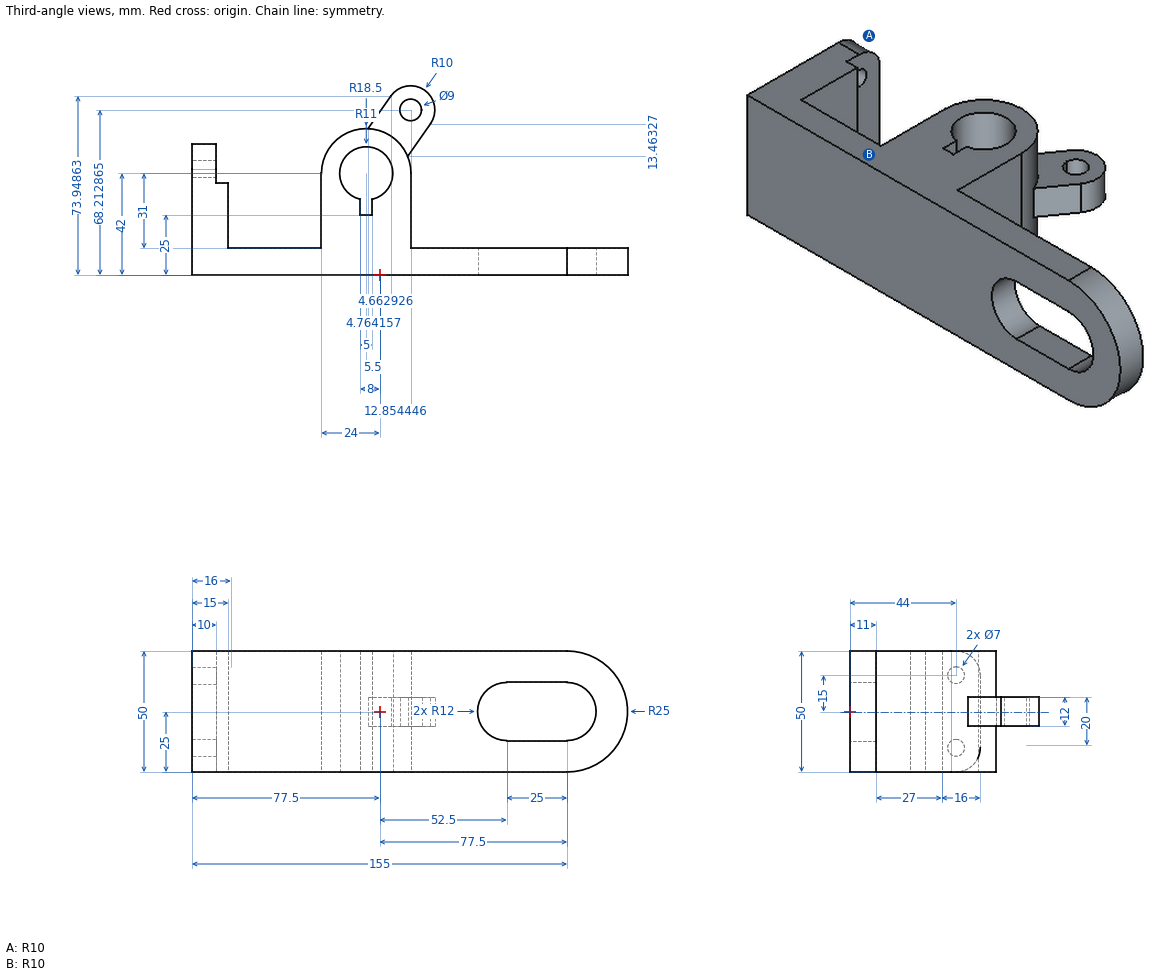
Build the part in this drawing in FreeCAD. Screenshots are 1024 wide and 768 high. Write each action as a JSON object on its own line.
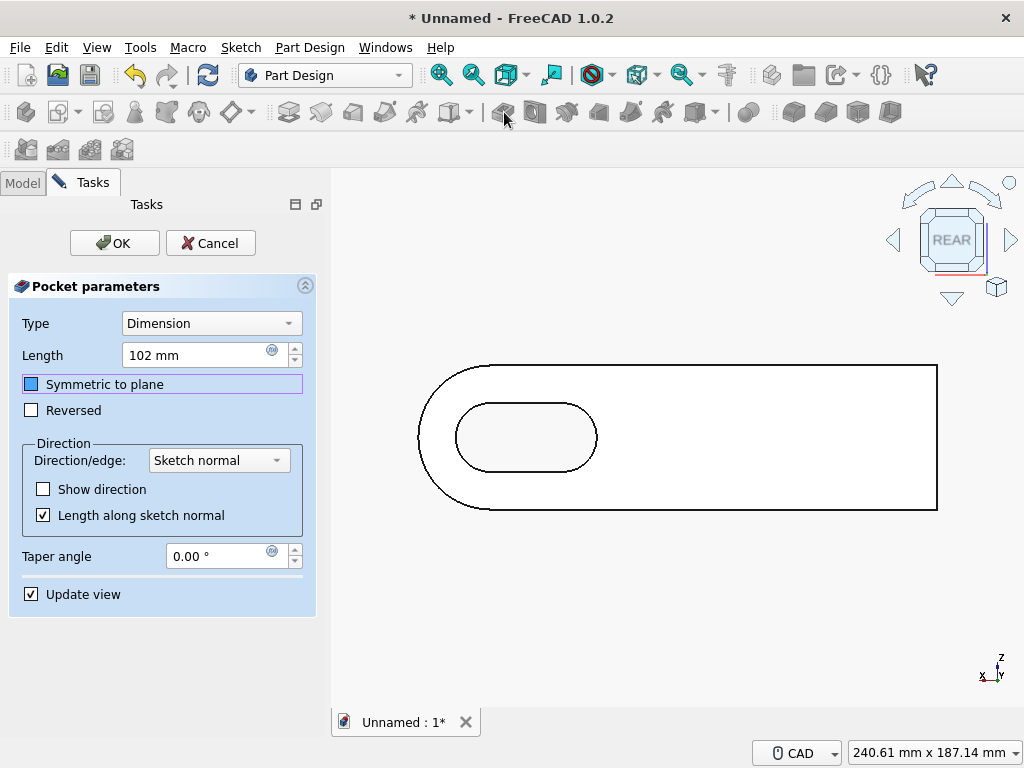
{"action": "left_click", "coordinate": [115, 243]}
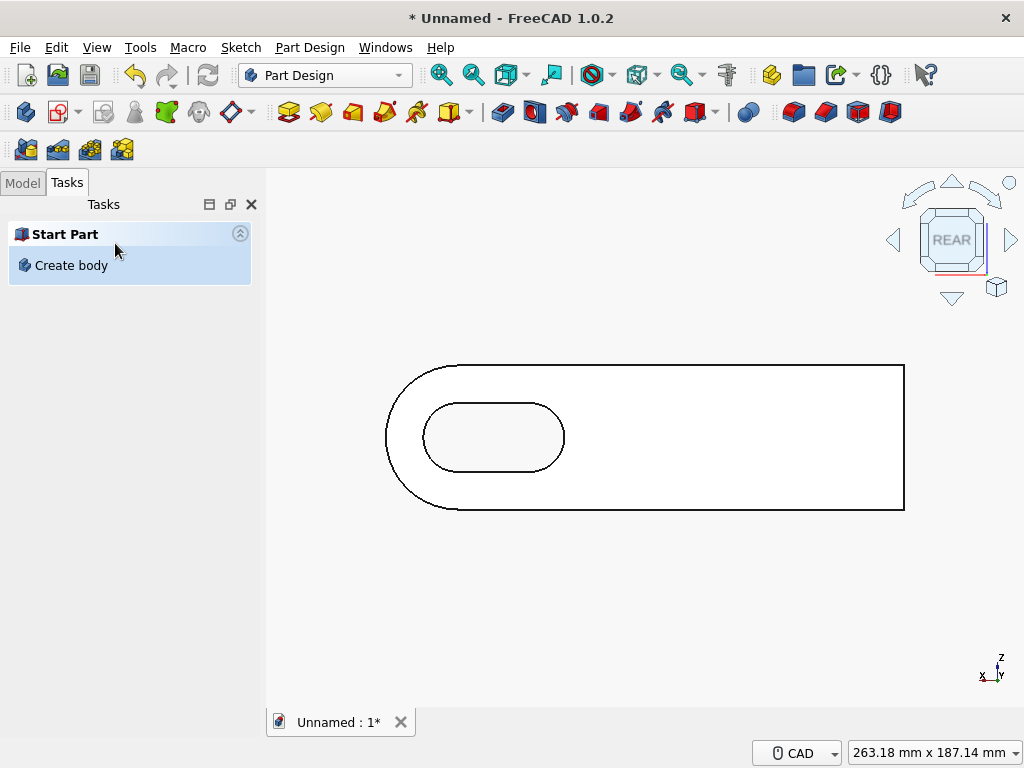
{"action": "key", "text": "0"}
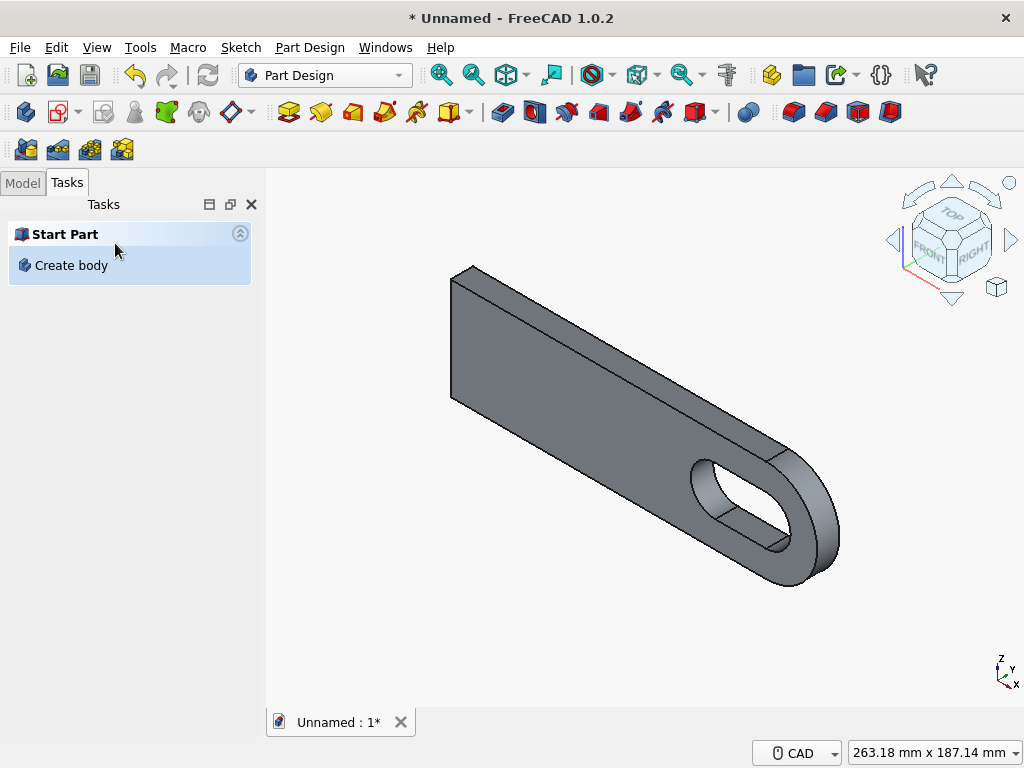
{"action": "left_click", "coordinate": [755, 441]}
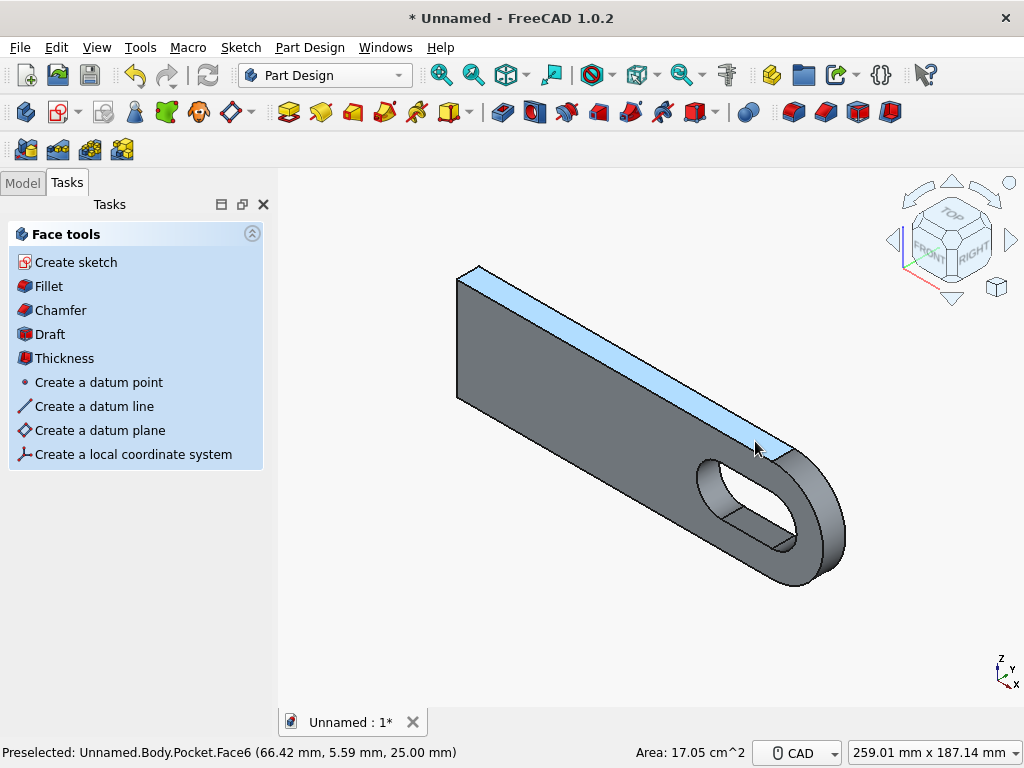
{"action": "left_click", "coordinate": [58, 112]}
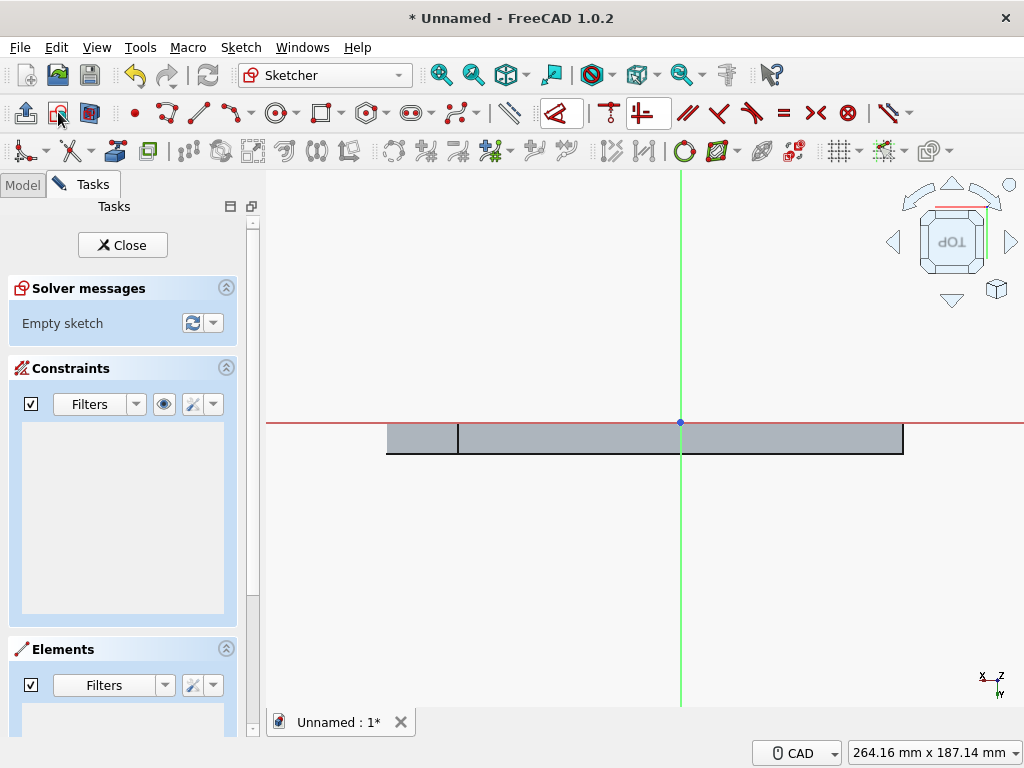
{"action": "scroll", "coordinate": [843, 596], "scroll_direction": "up", "scroll_amount": 3}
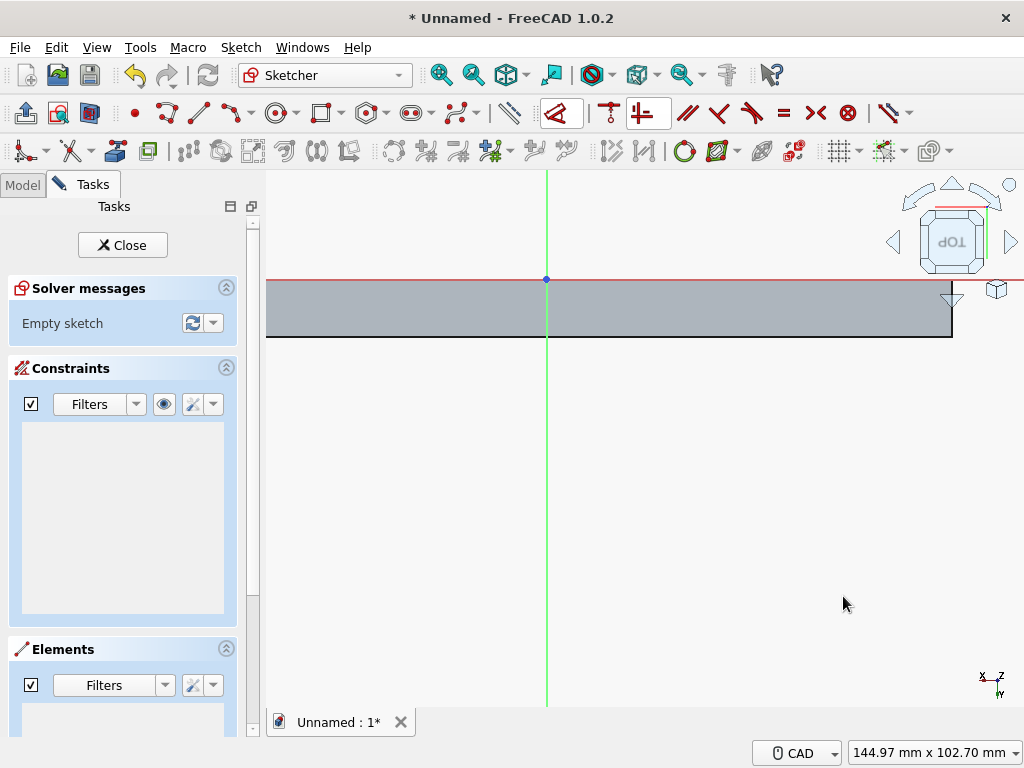
{"action": "left_click", "coordinate": [168, 114]}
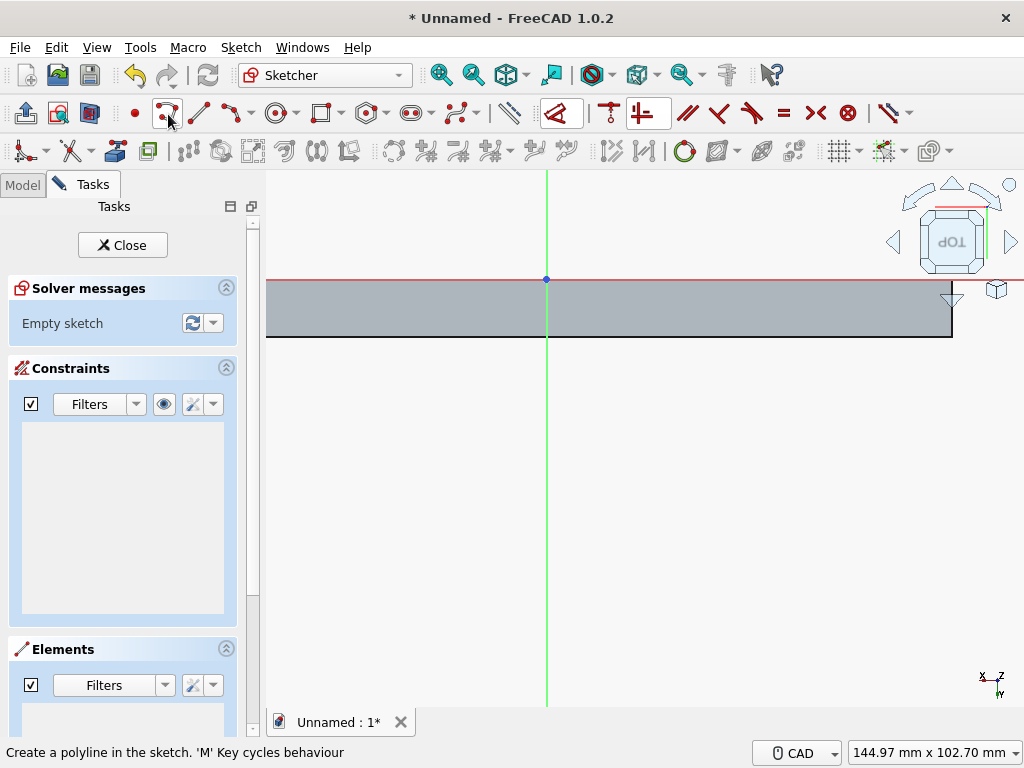
{"action": "left_click", "coordinate": [672, 499]}
{"action": "left_click", "coordinate": [672, 337]}
{"action": "left_click", "coordinate": [479, 337]}
{"action": "left_click", "coordinate": [479, 499]}
{"action": "right_click", "coordinate": [479, 499]}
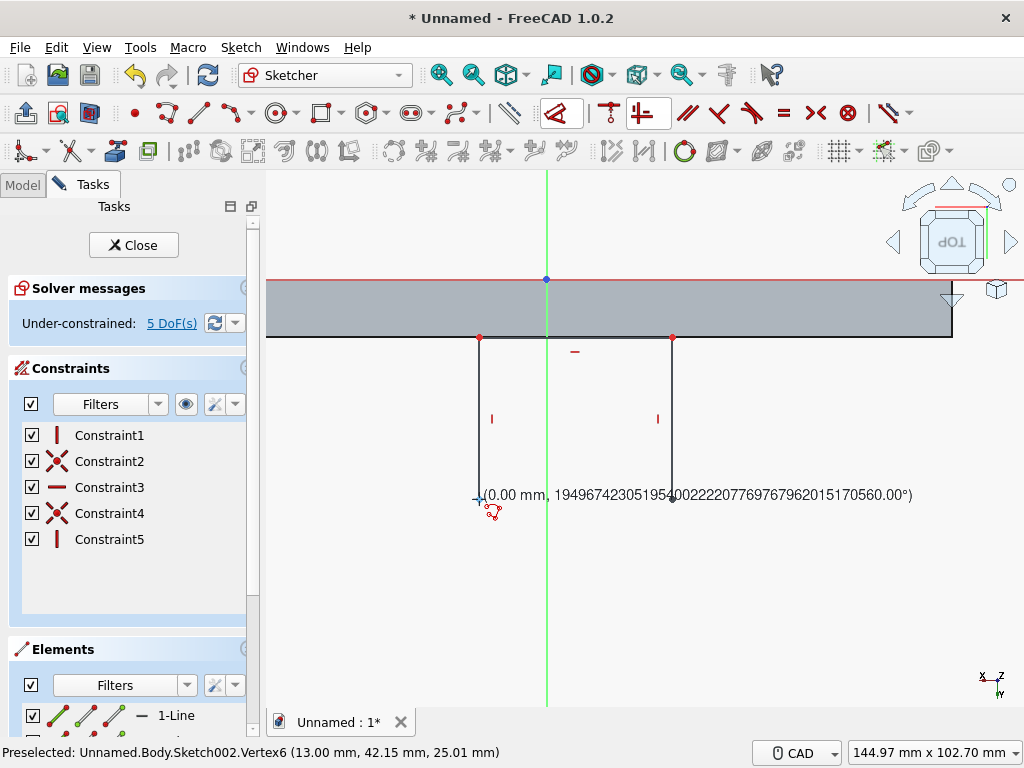
{"action": "left_click", "coordinate": [232, 114]}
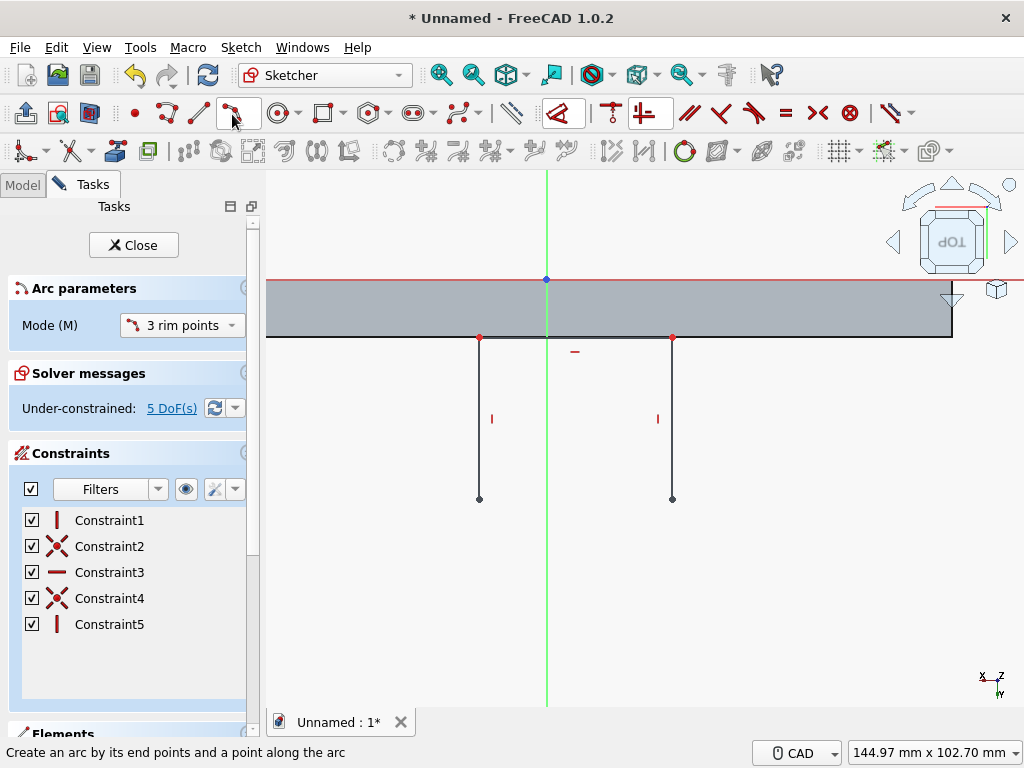
{"action": "left_click", "coordinate": [479, 500]}
{"action": "left_click", "coordinate": [672, 500]}
{"action": "left_click", "coordinate": [576, 596]}
{"action": "key", "text": "Escape"}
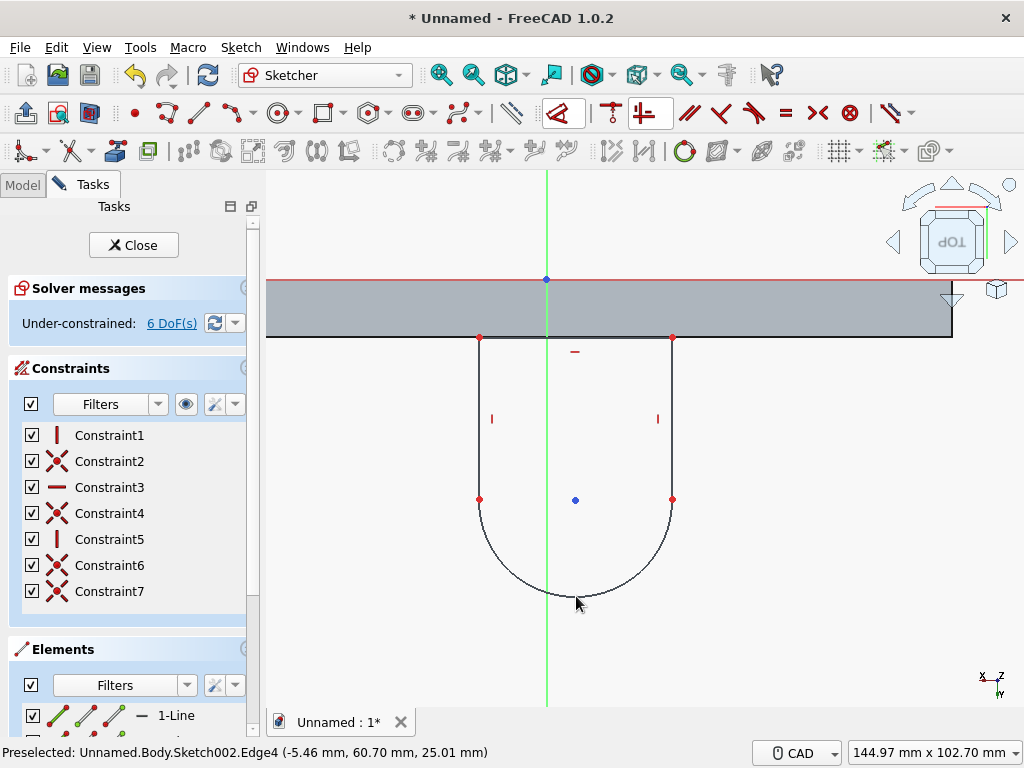
{"action": "left_click", "coordinate": [672, 451]}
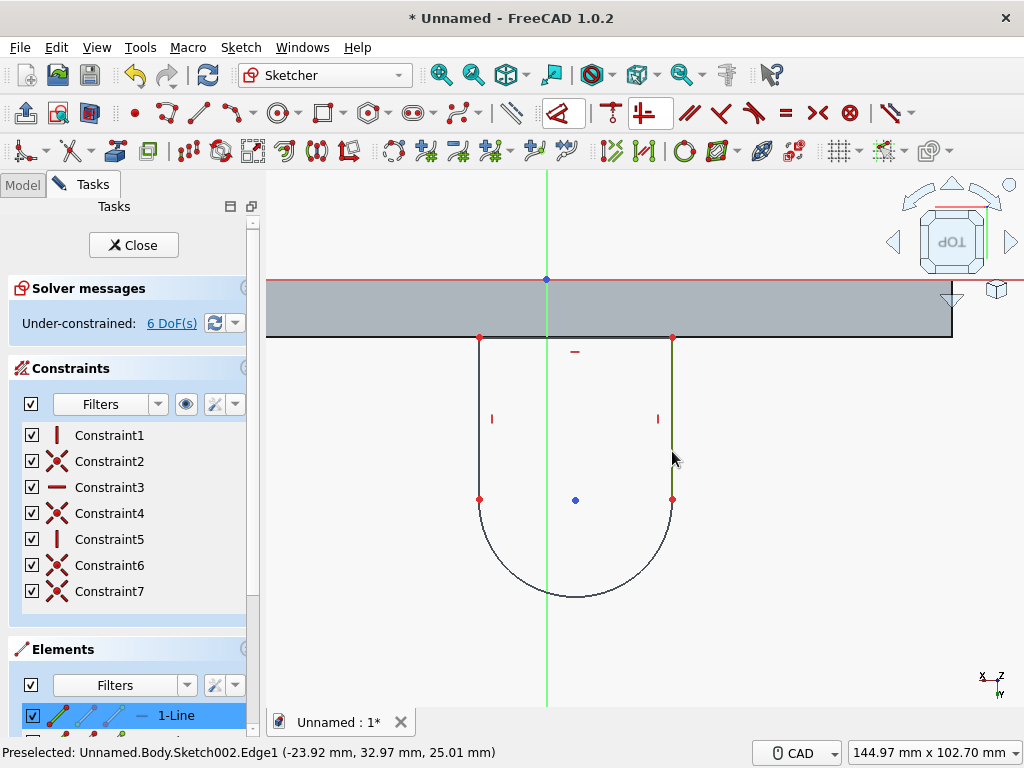
{"action": "left_click", "coordinate": [519, 578]}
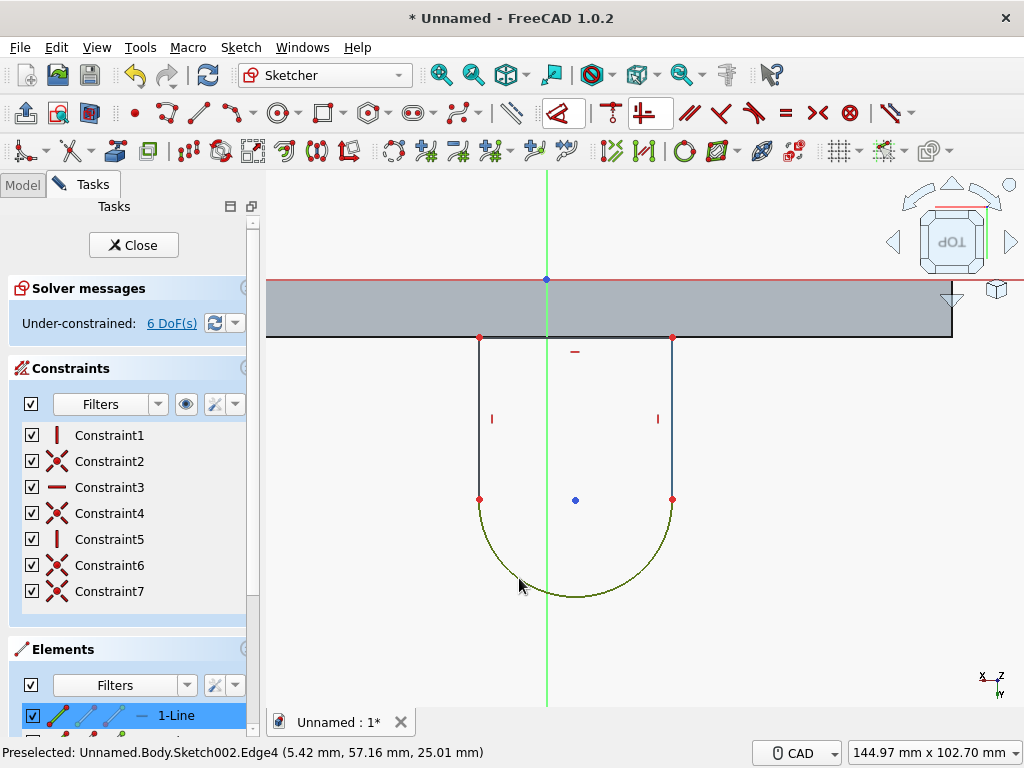
{"action": "left_click", "coordinate": [754, 114]}